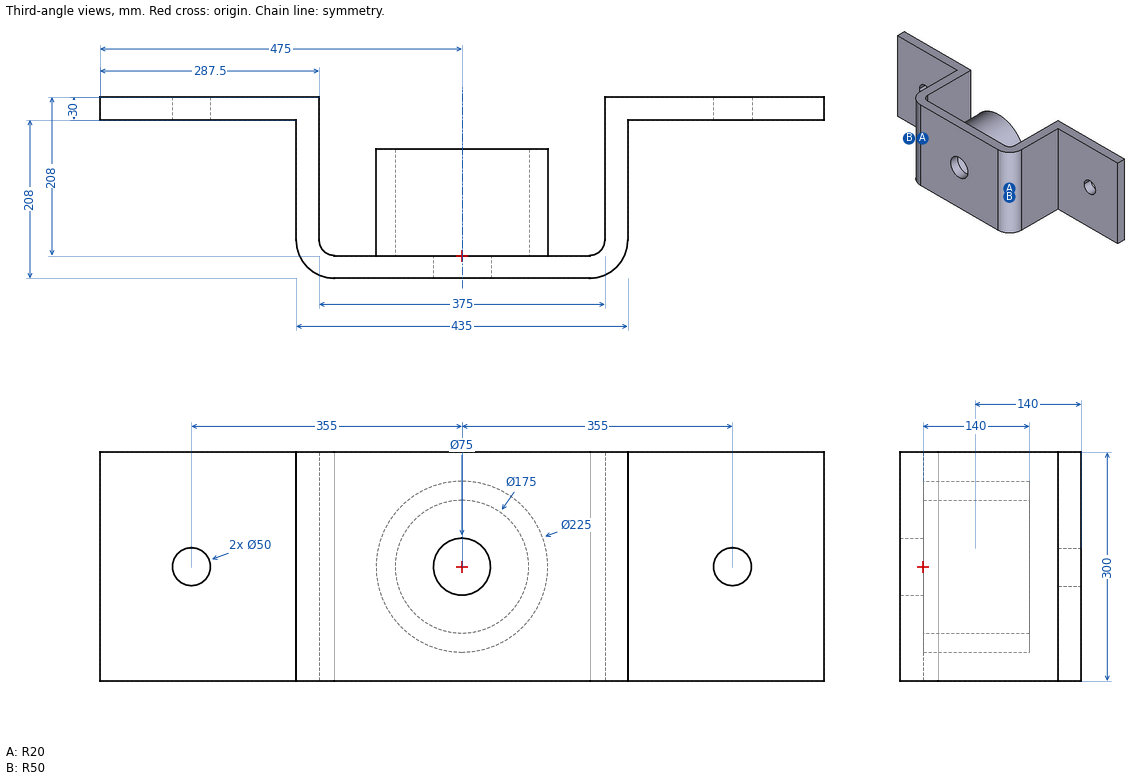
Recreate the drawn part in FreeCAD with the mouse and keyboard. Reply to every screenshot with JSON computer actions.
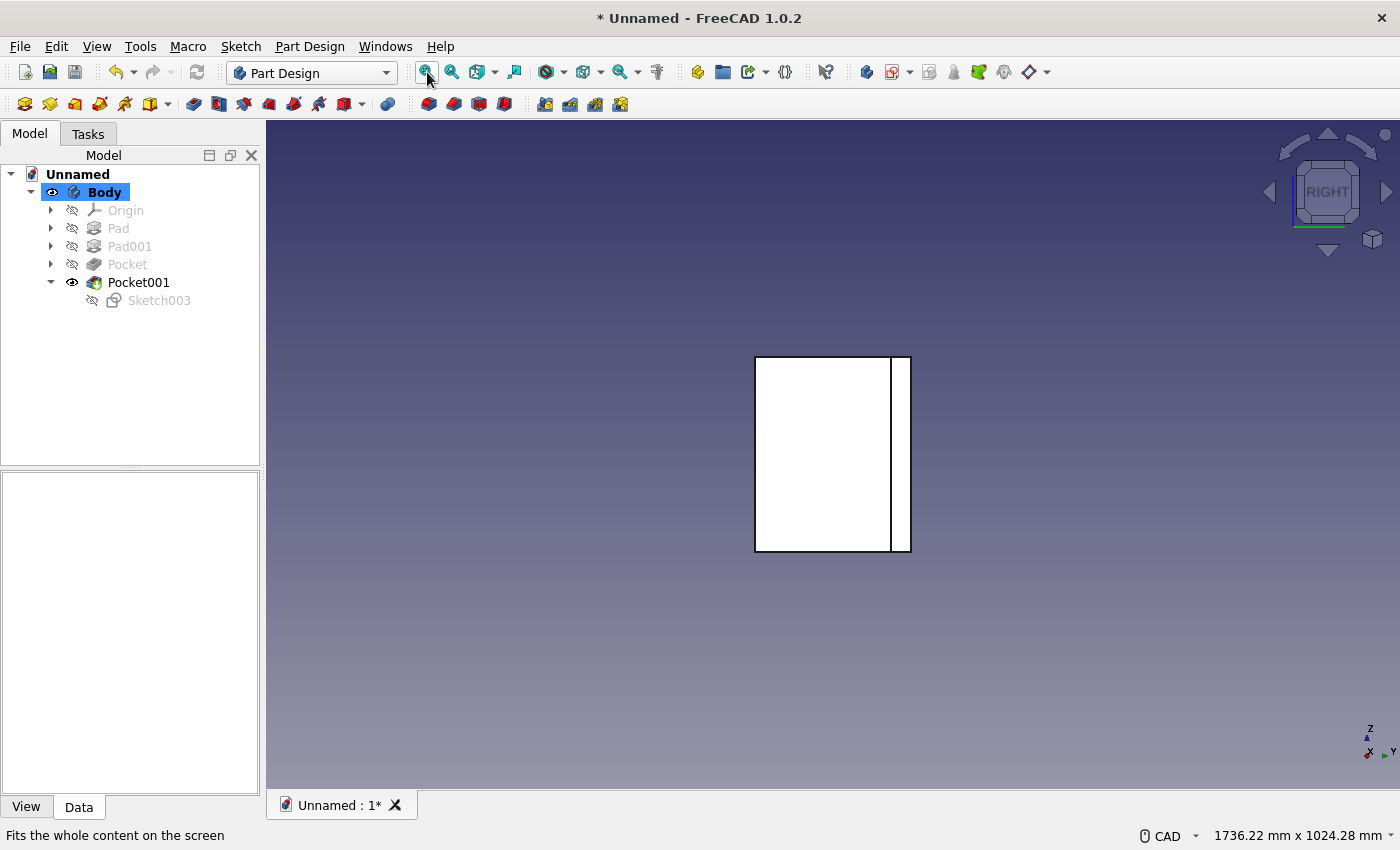
{"action": "key", "text": "5"}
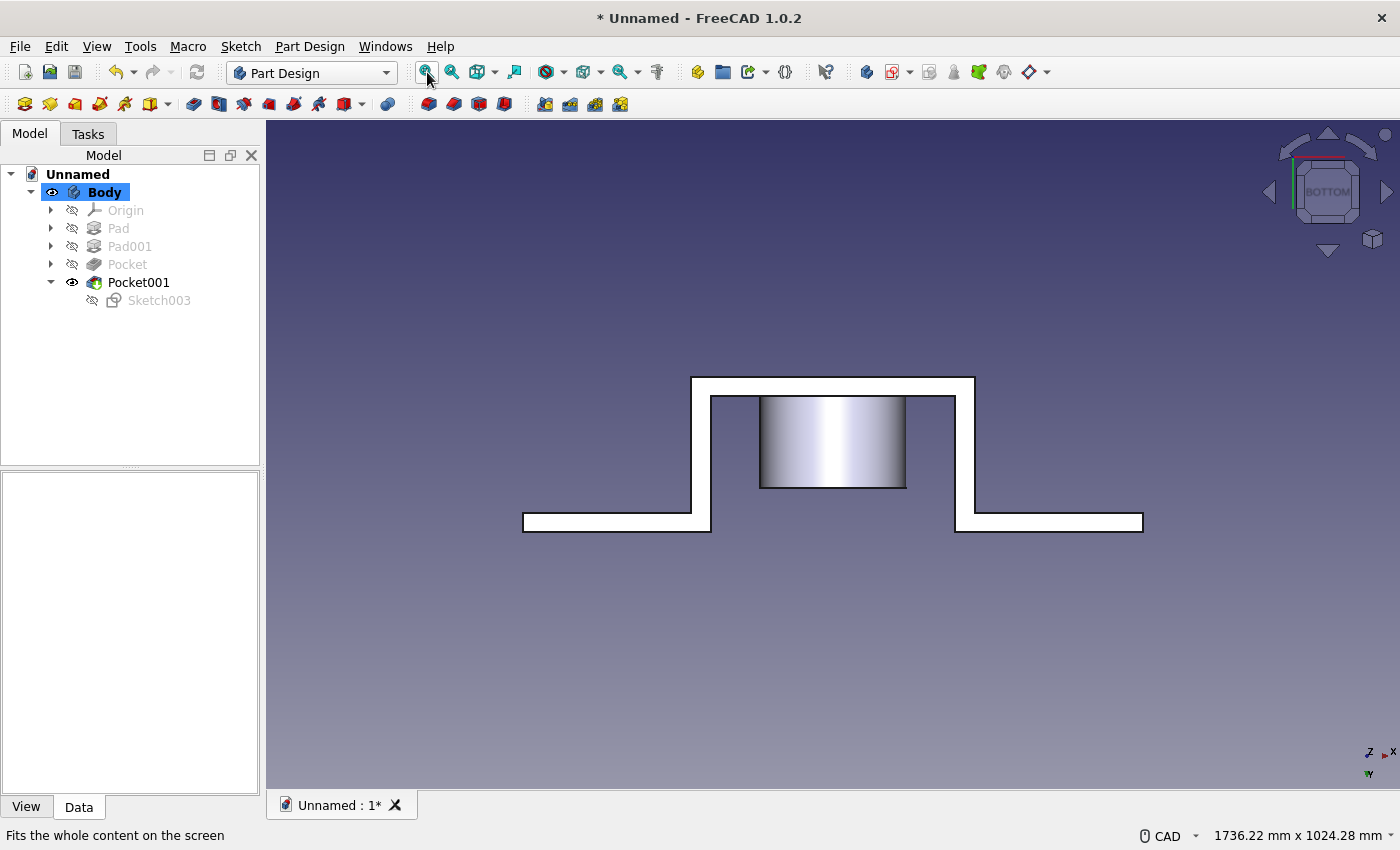
{"action": "key", "text": "4"}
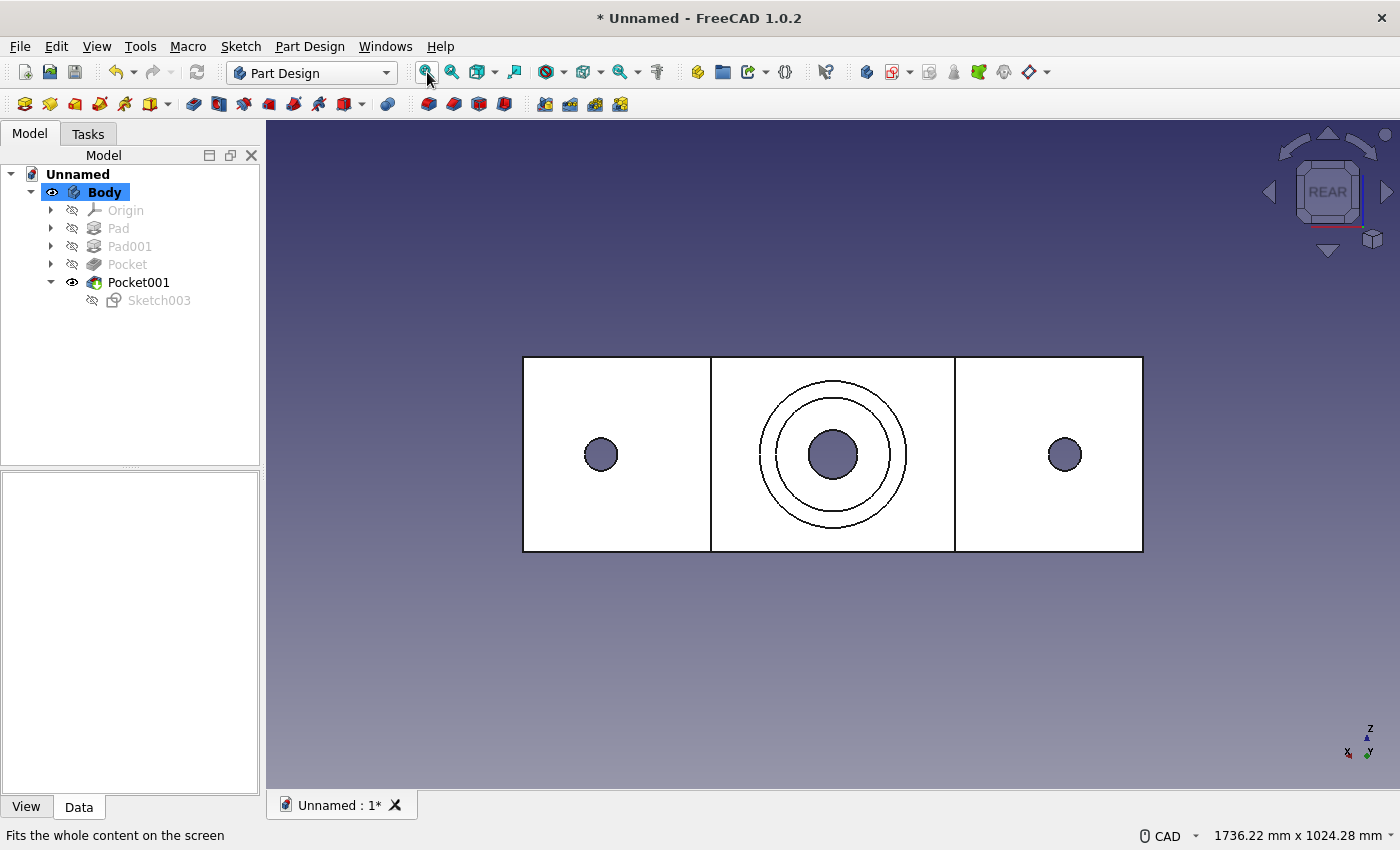
{"action": "key", "text": "6"}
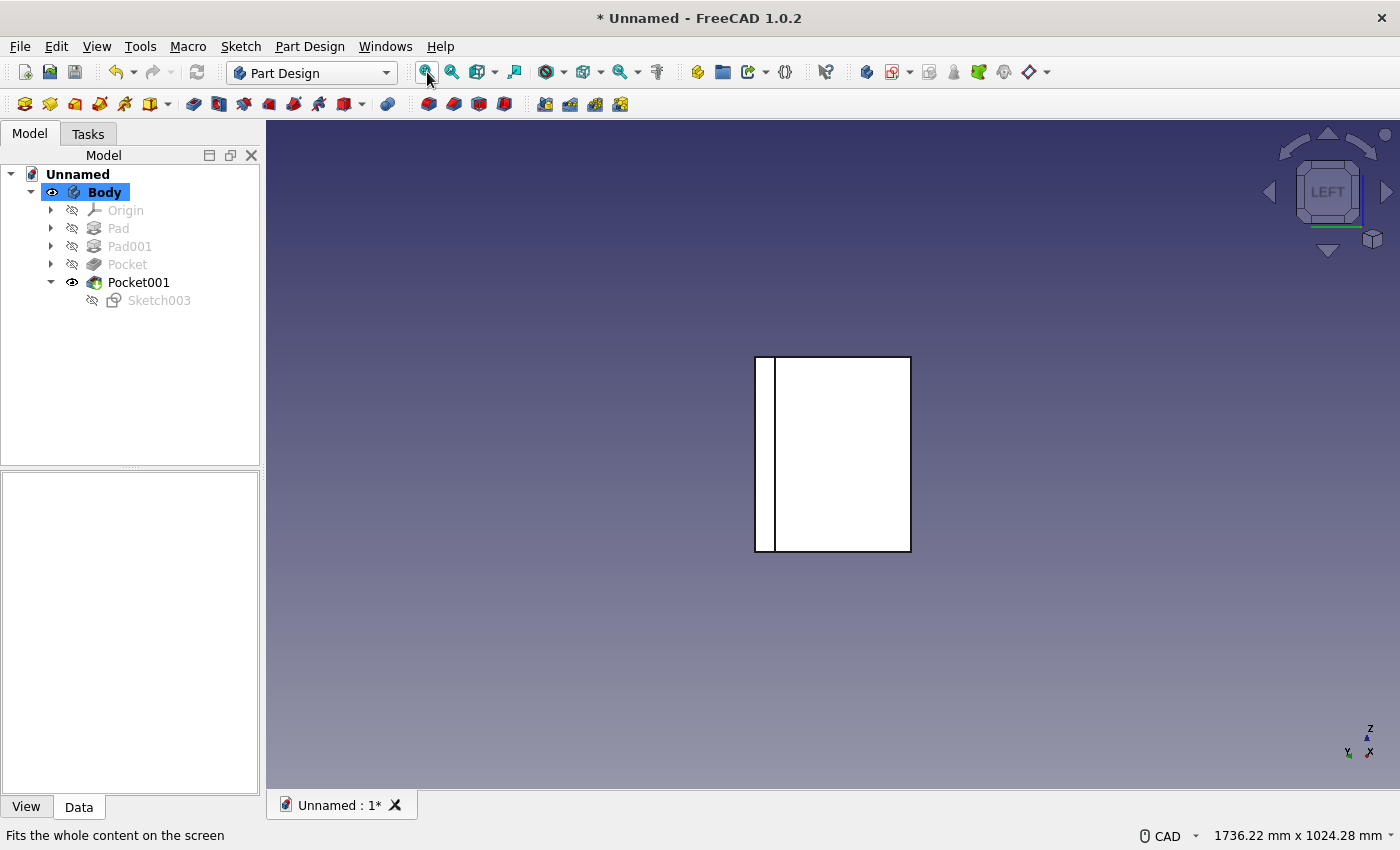
{"action": "left_click", "coordinate": [427, 72]}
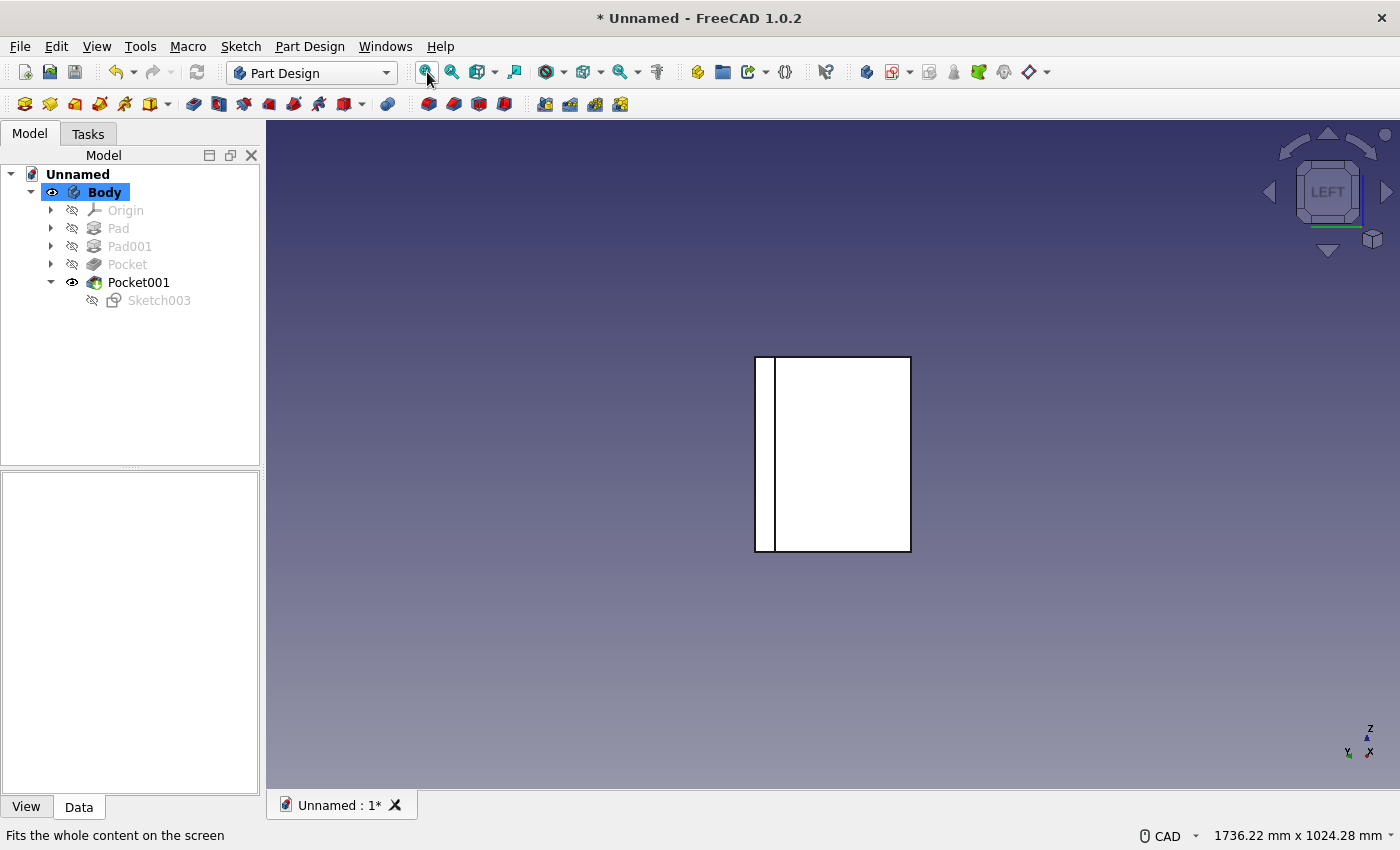
{"action": "key", "text": "v 3"}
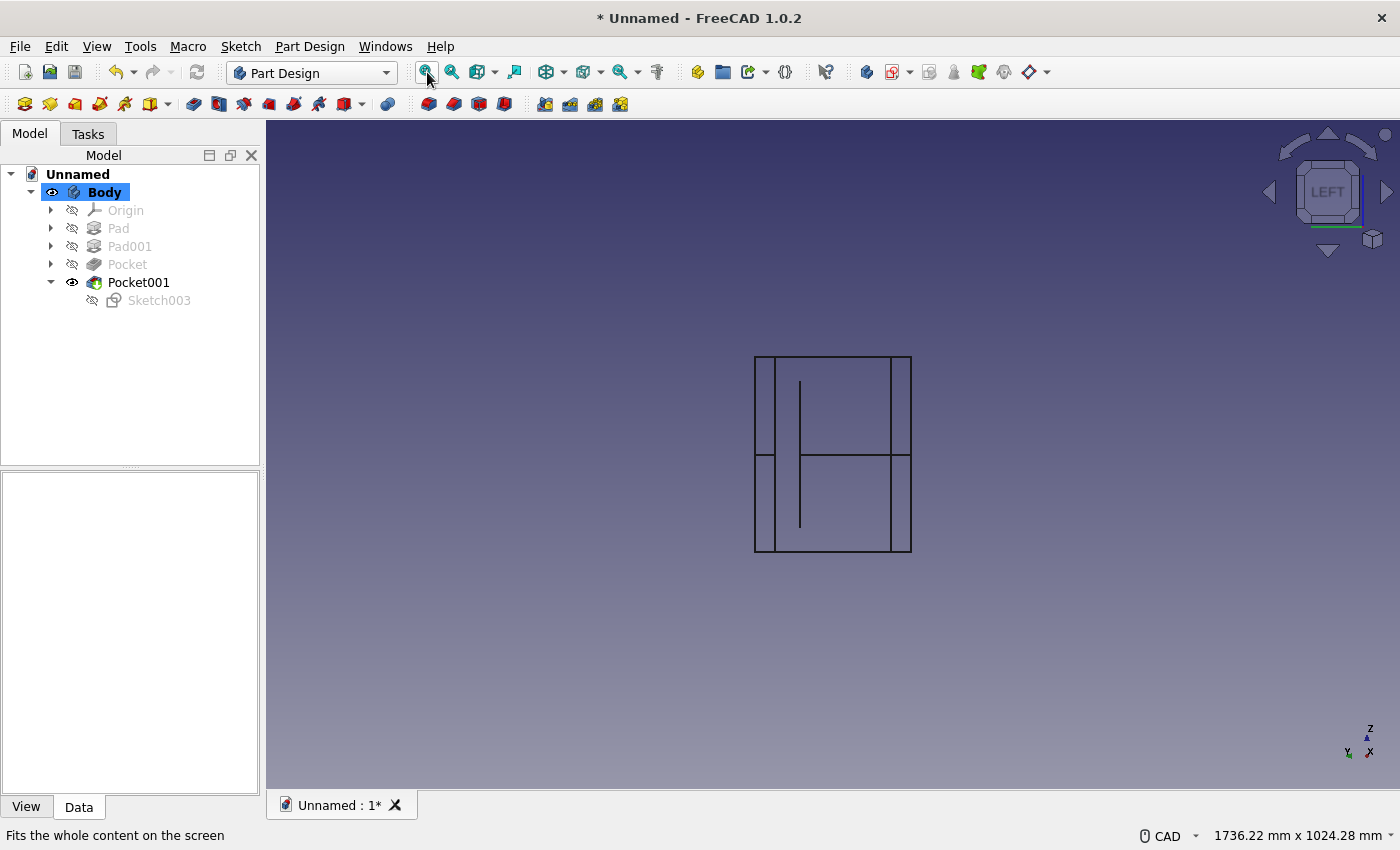
{"action": "key", "text": "0"}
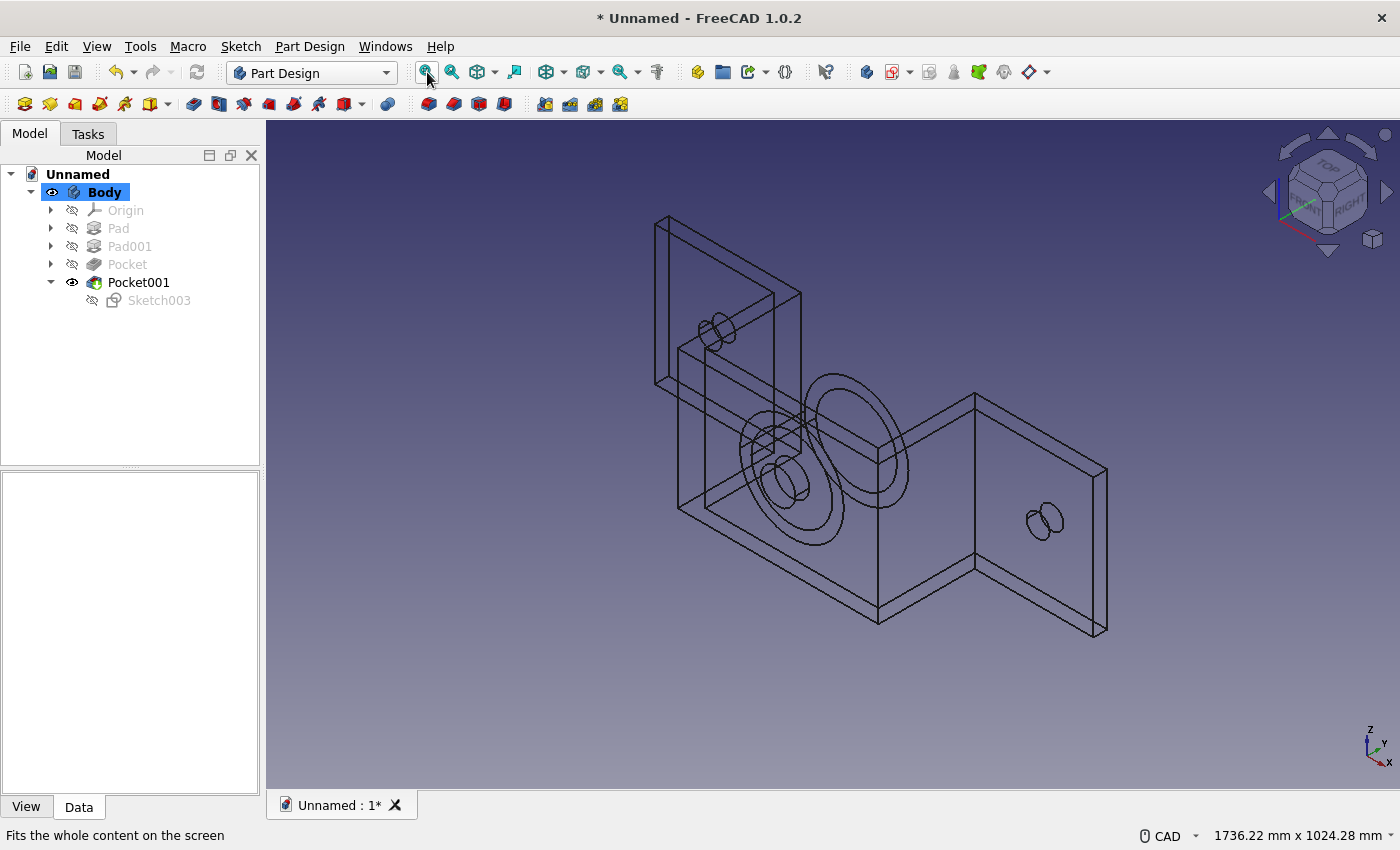
{"action": "left_click", "coordinate": [705, 427]}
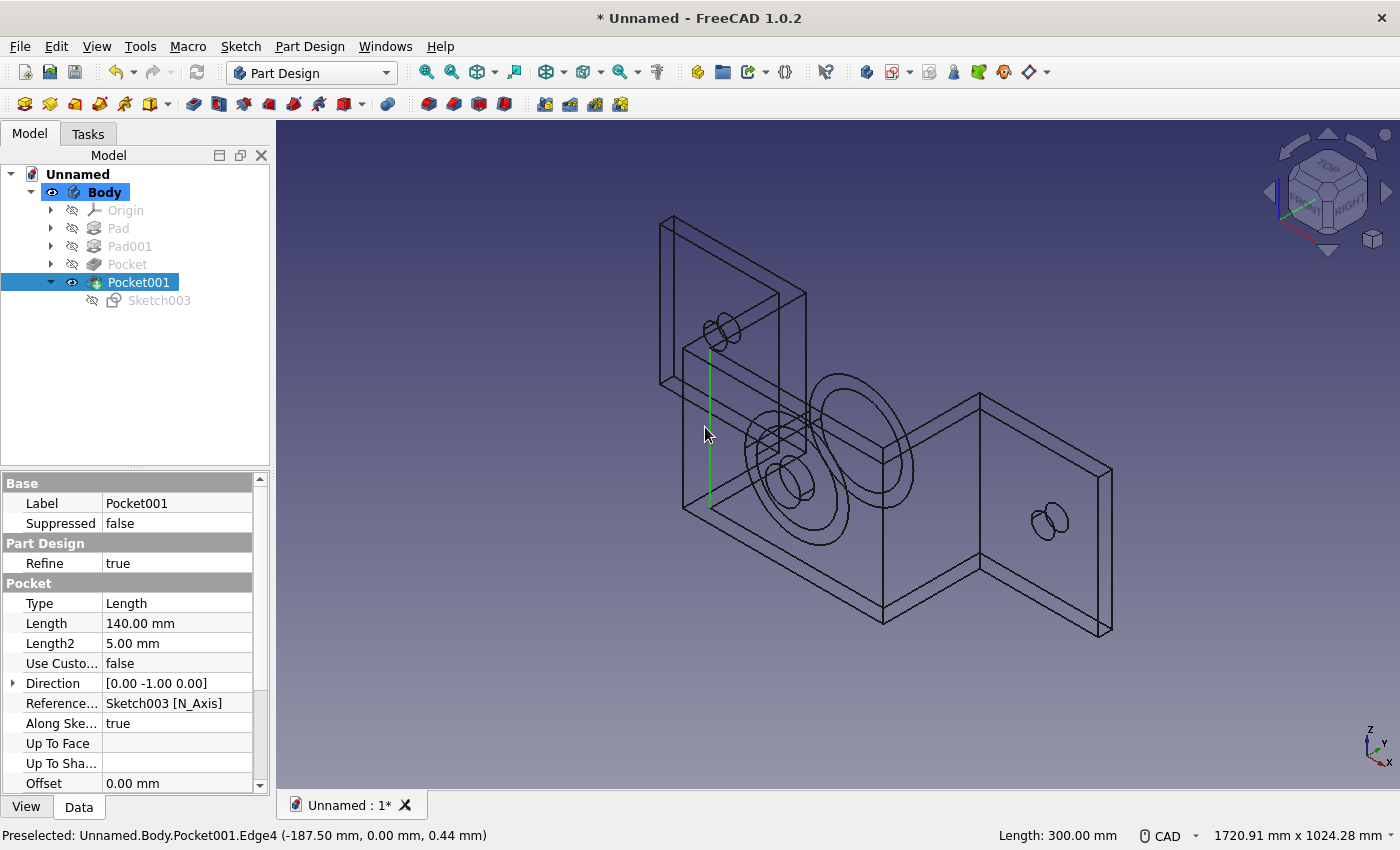
{"action": "key", "text": "2"}